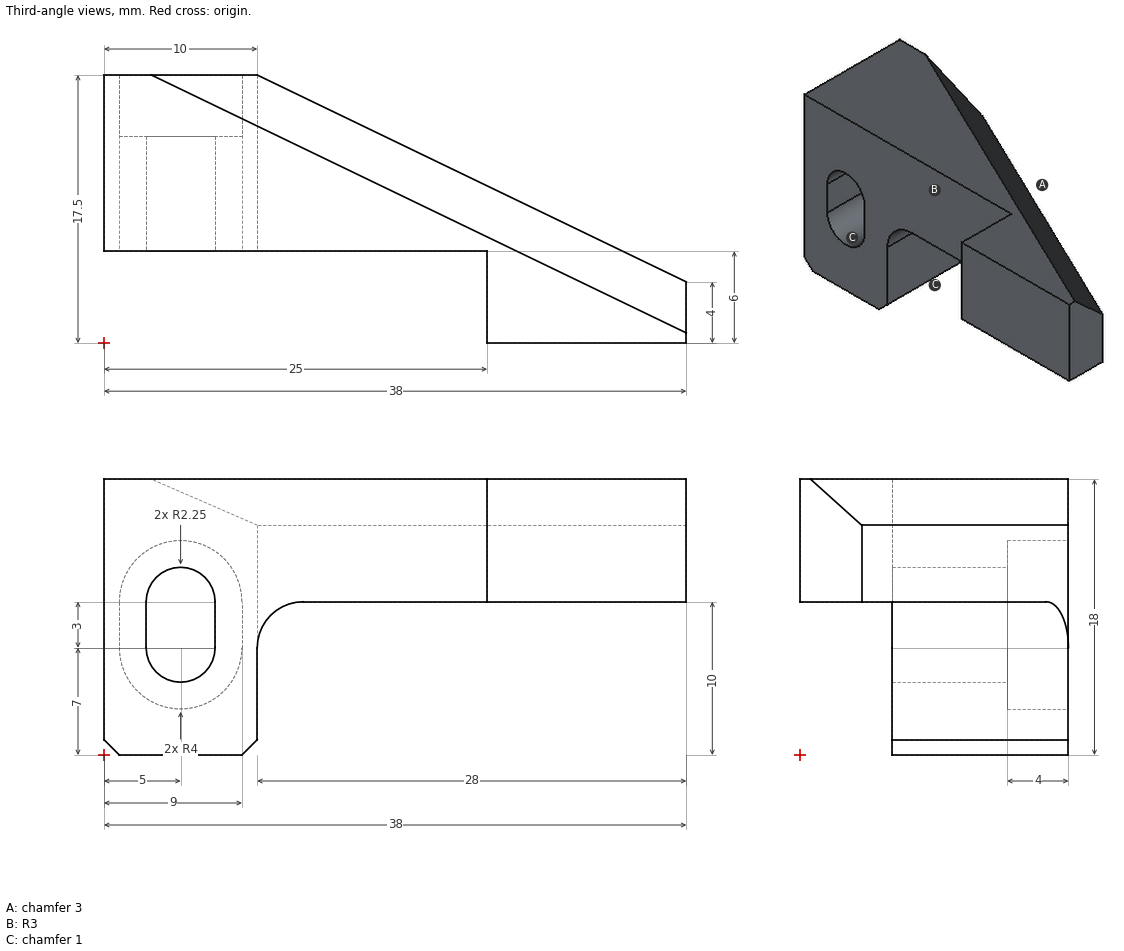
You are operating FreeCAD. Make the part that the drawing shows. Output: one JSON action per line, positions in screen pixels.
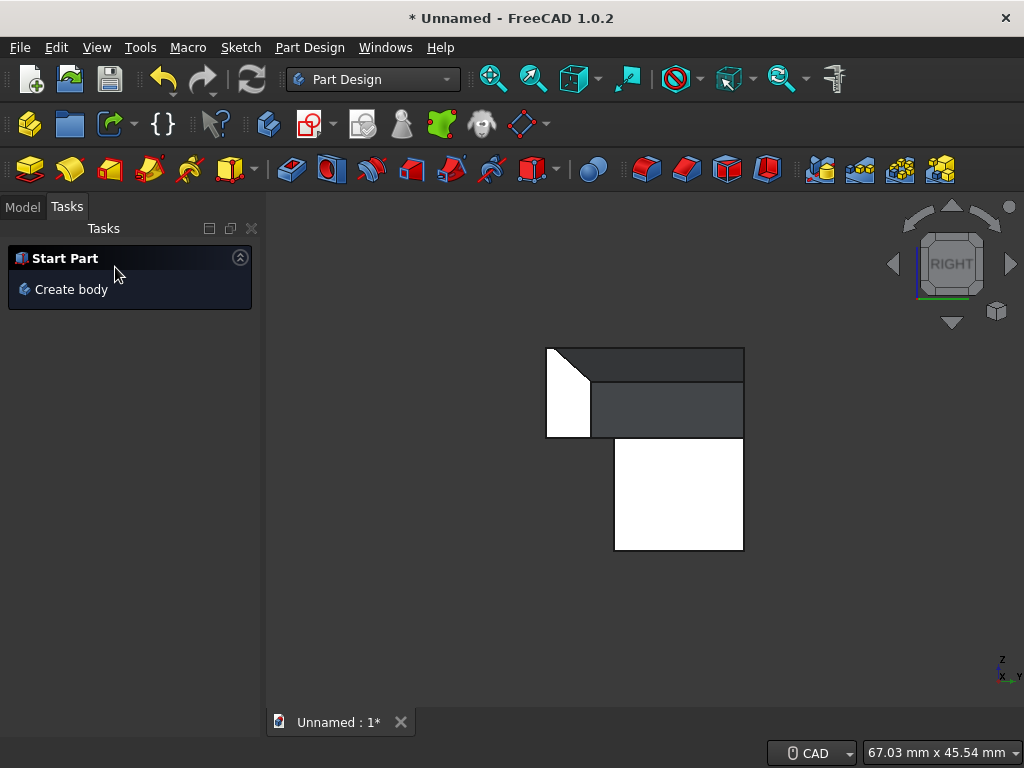
{"action": "key", "text": "5"}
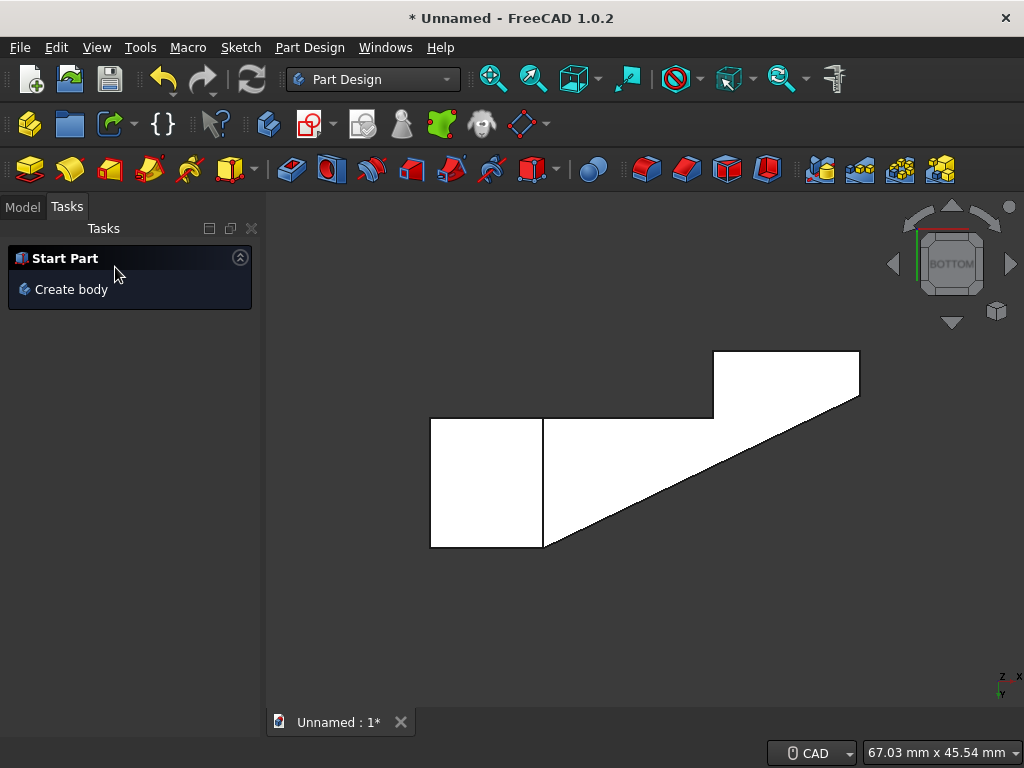
{"action": "key", "text": "4"}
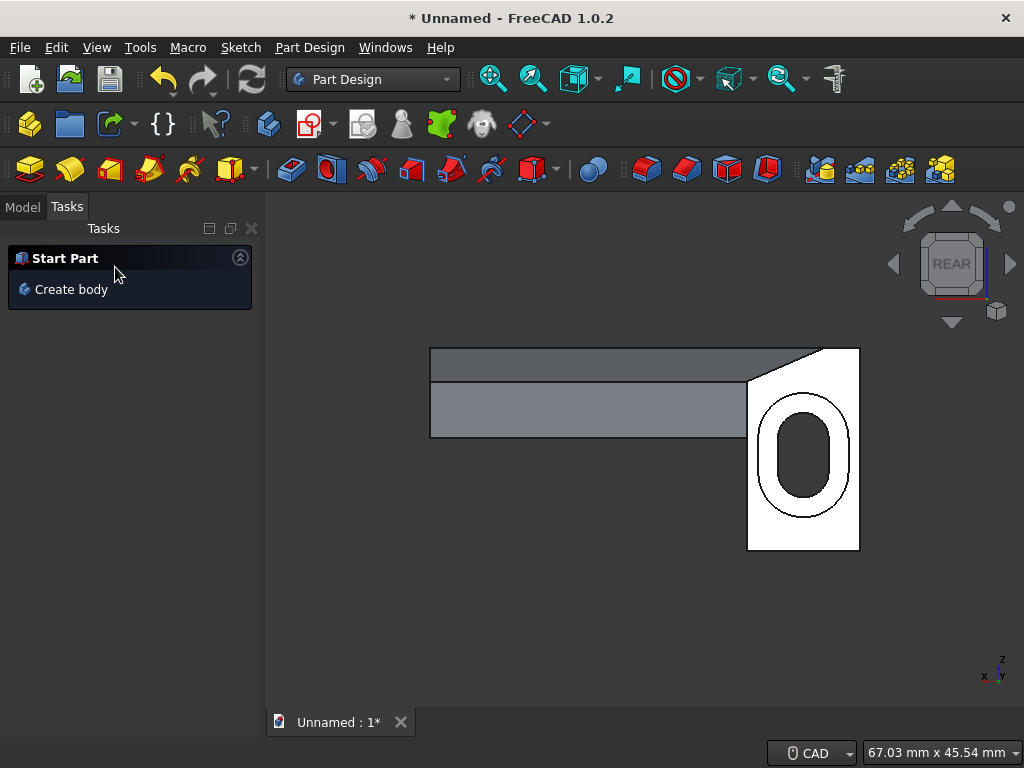
{"action": "key", "text": "6"}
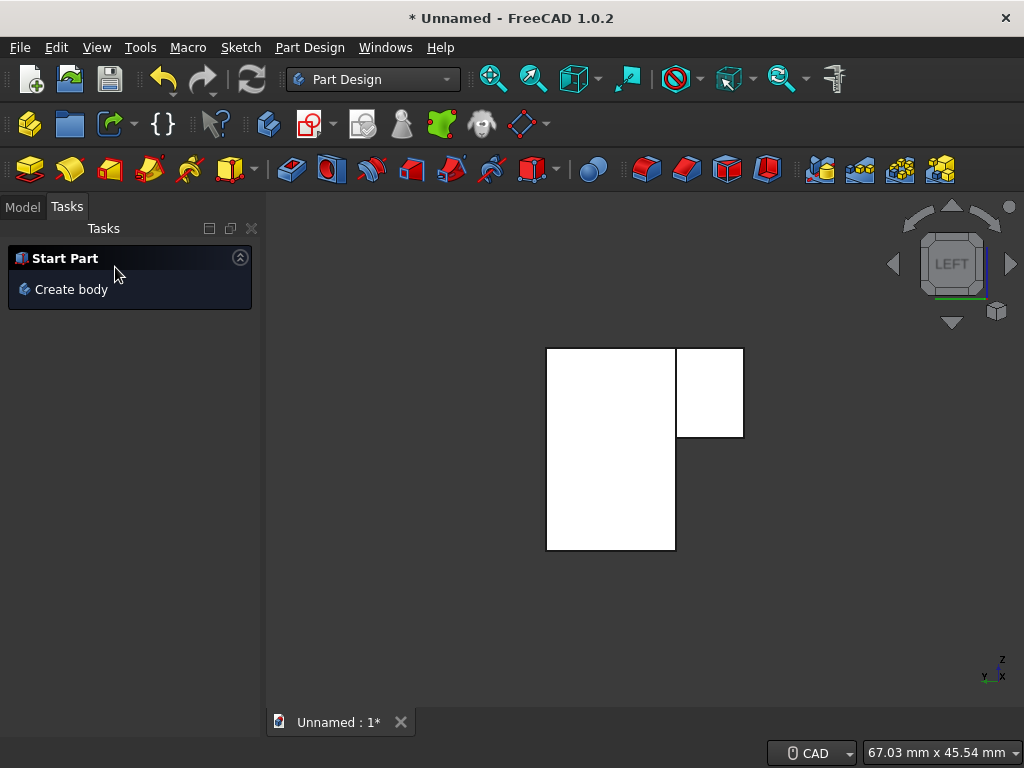
{"action": "left_click", "coordinate": [494, 80]}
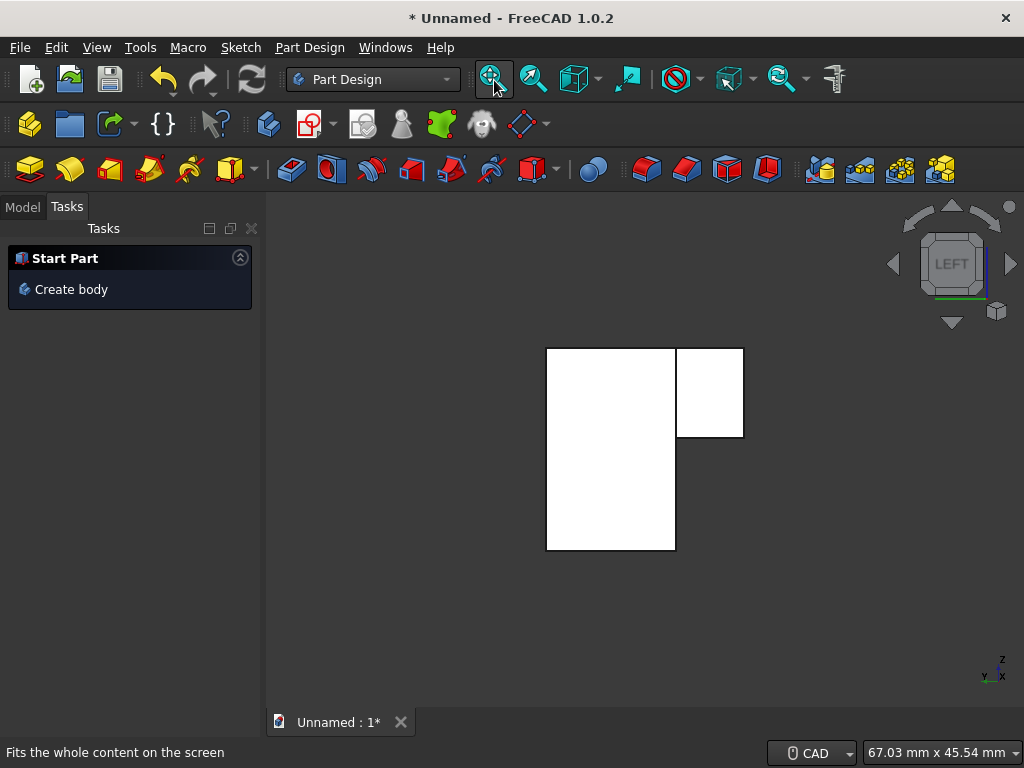
{"action": "key", "text": "v 3"}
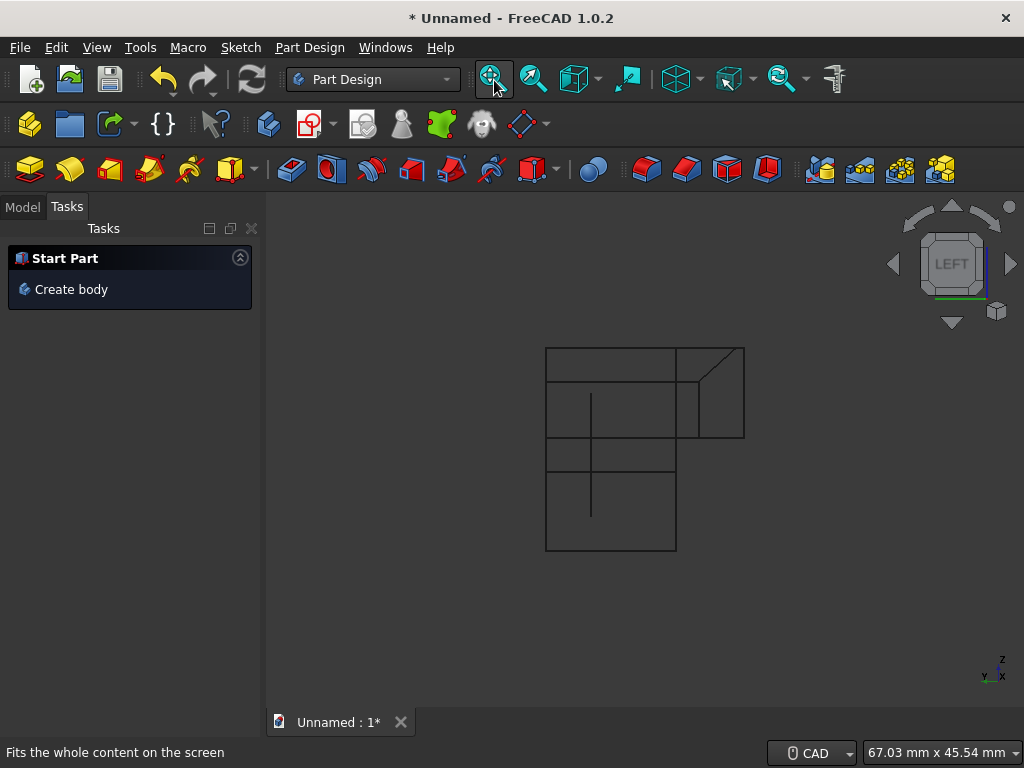
{"action": "key", "text": "0"}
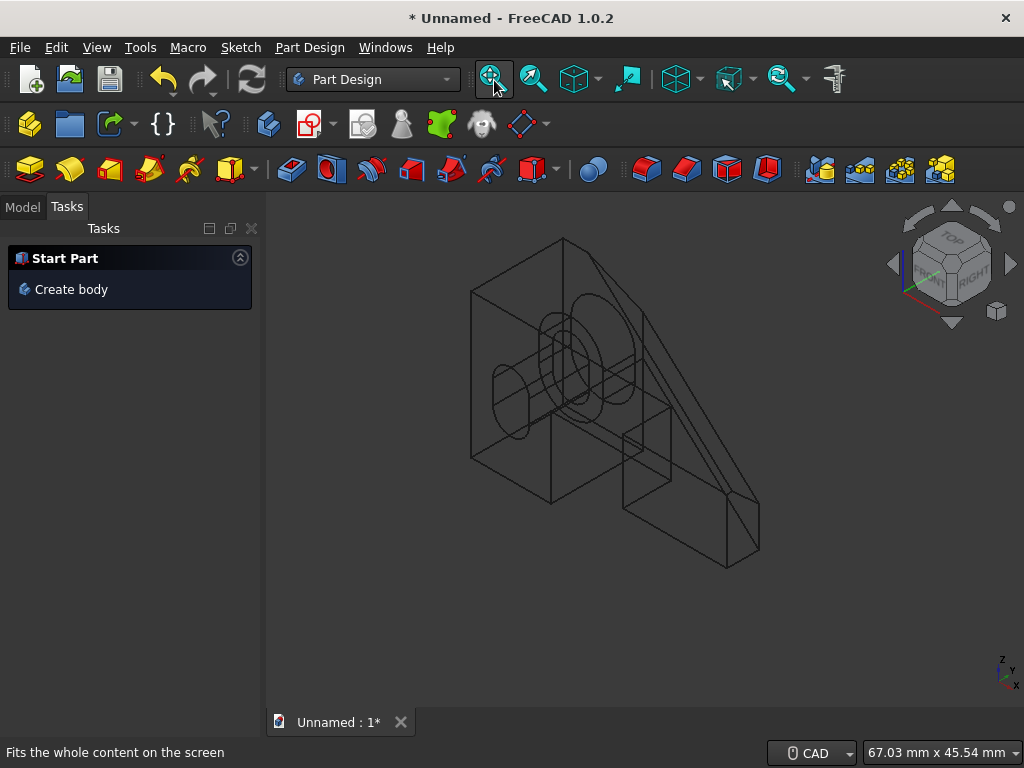
{"action": "left_click", "coordinate": [597, 384]}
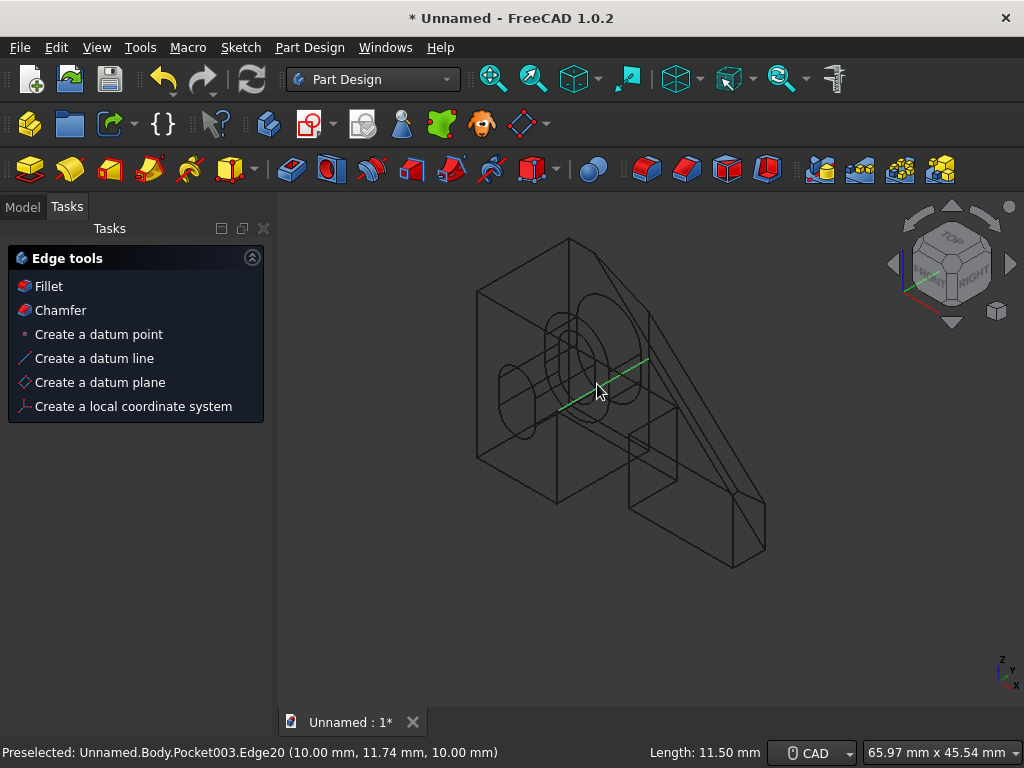
{"action": "key", "text": "v 1"}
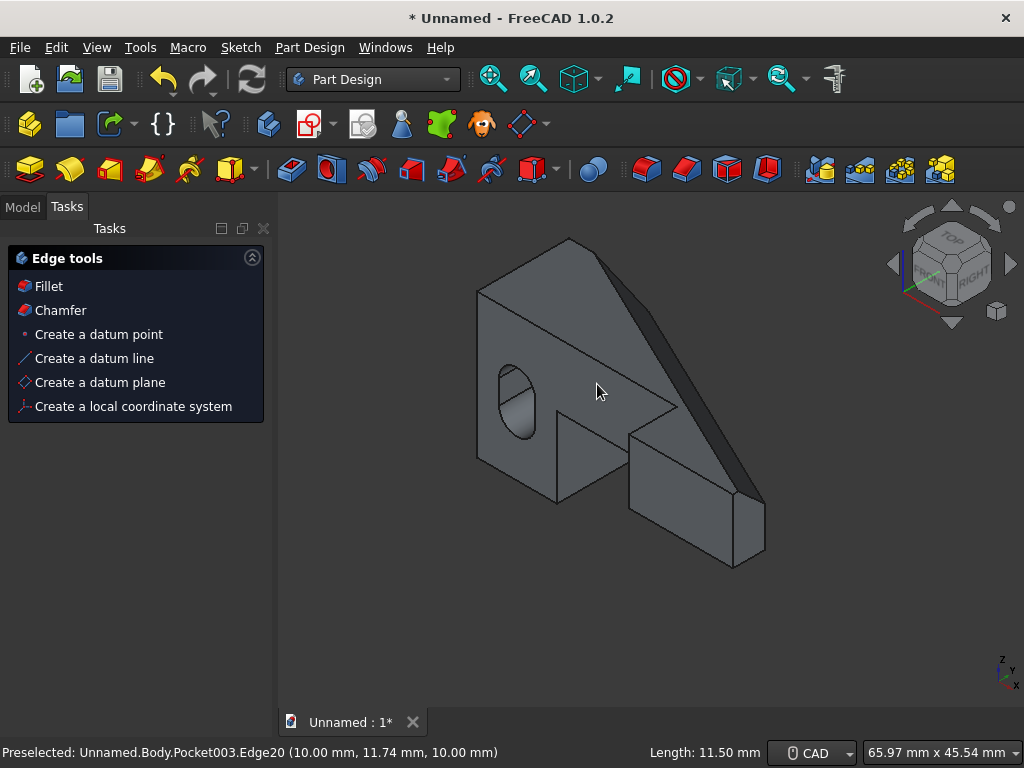
{"action": "left_click", "coordinate": [648, 170]}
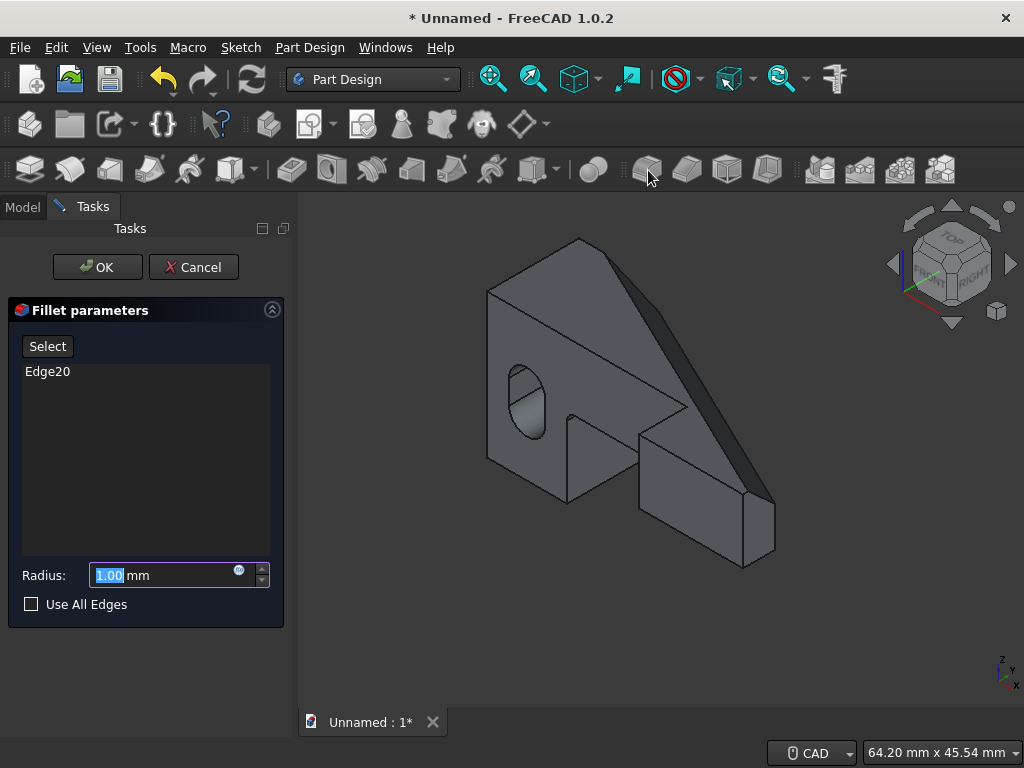
{"action": "type", "text": "3"}
{"action": "key", "text": "Tab"}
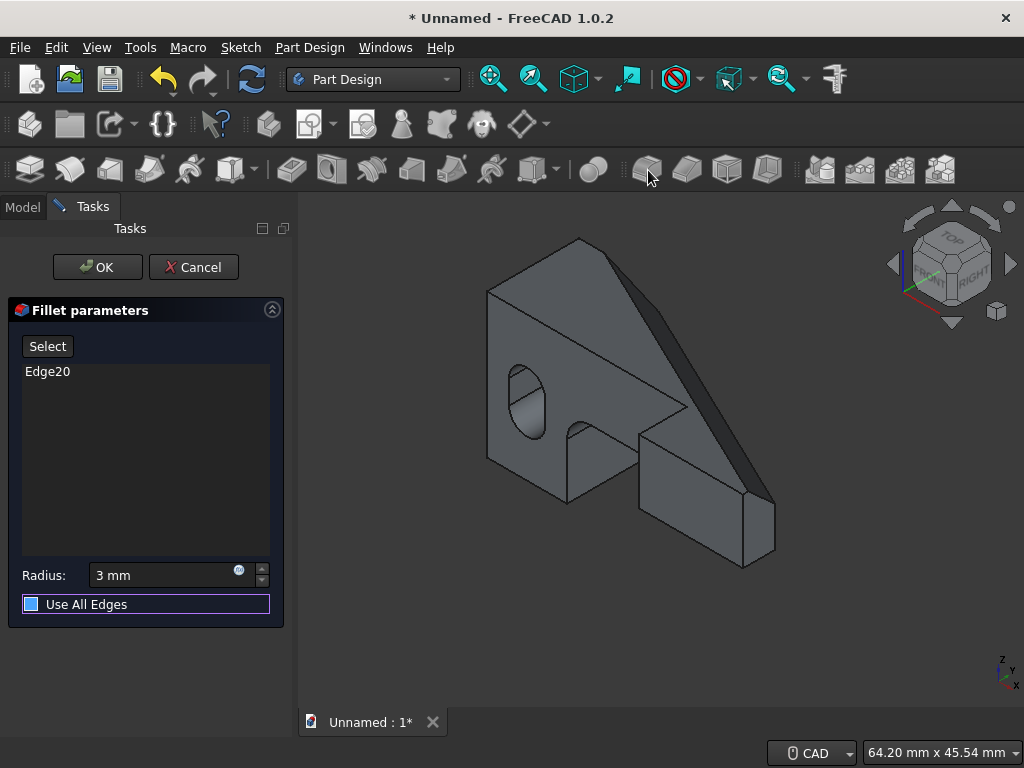
{"action": "left_click", "coordinate": [98, 267]}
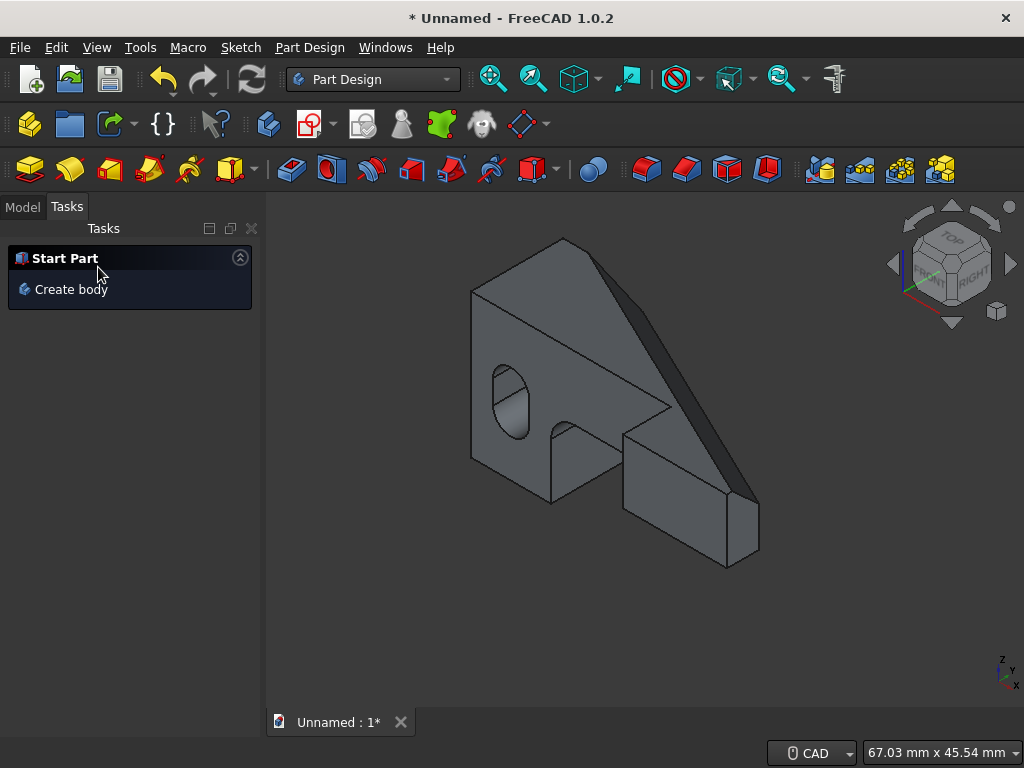
{"action": "key", "text": "2"}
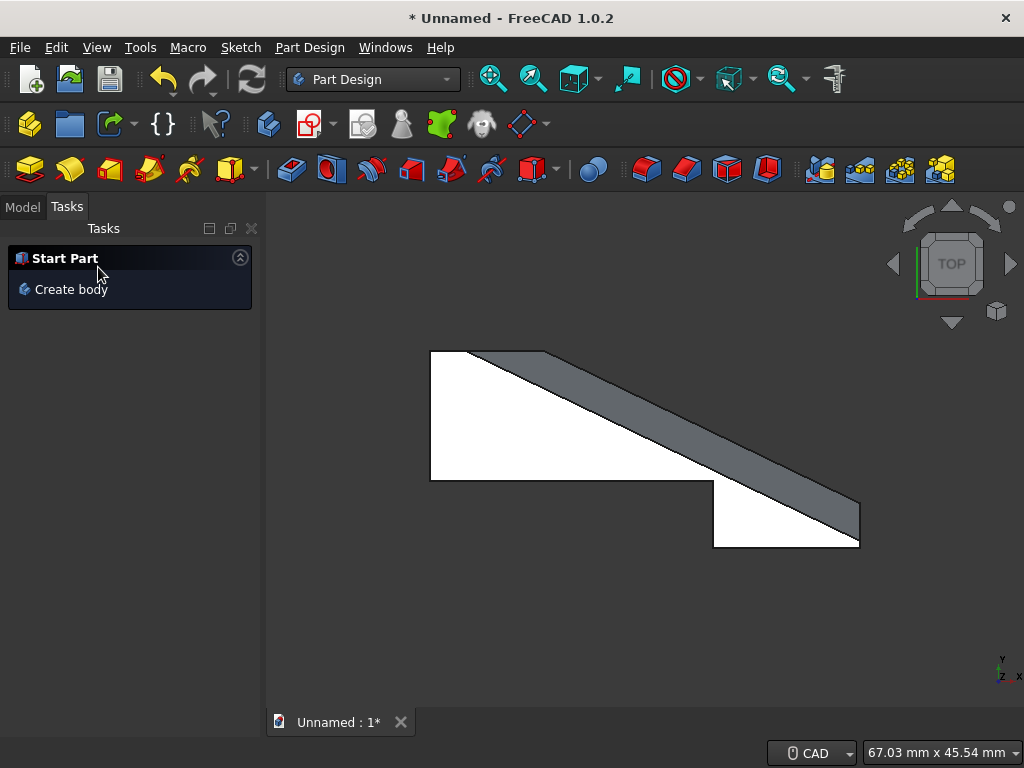
{"action": "key", "text": "0"}